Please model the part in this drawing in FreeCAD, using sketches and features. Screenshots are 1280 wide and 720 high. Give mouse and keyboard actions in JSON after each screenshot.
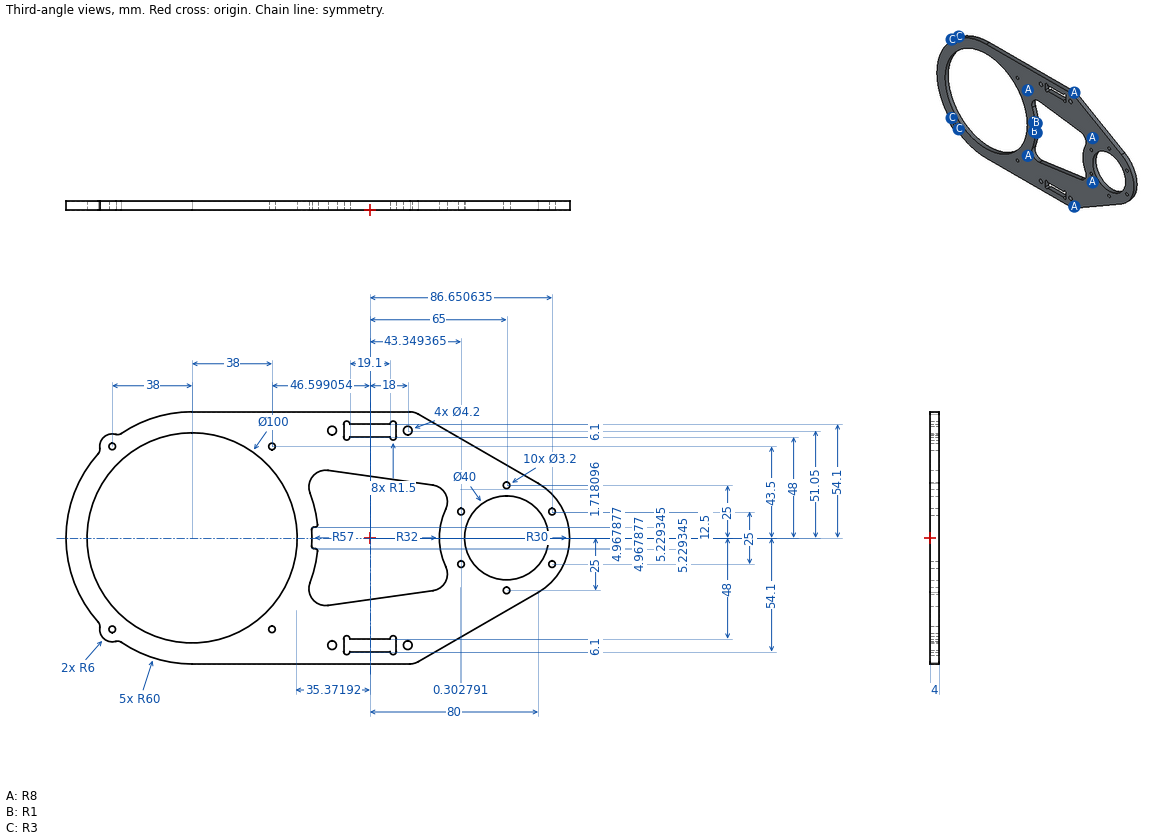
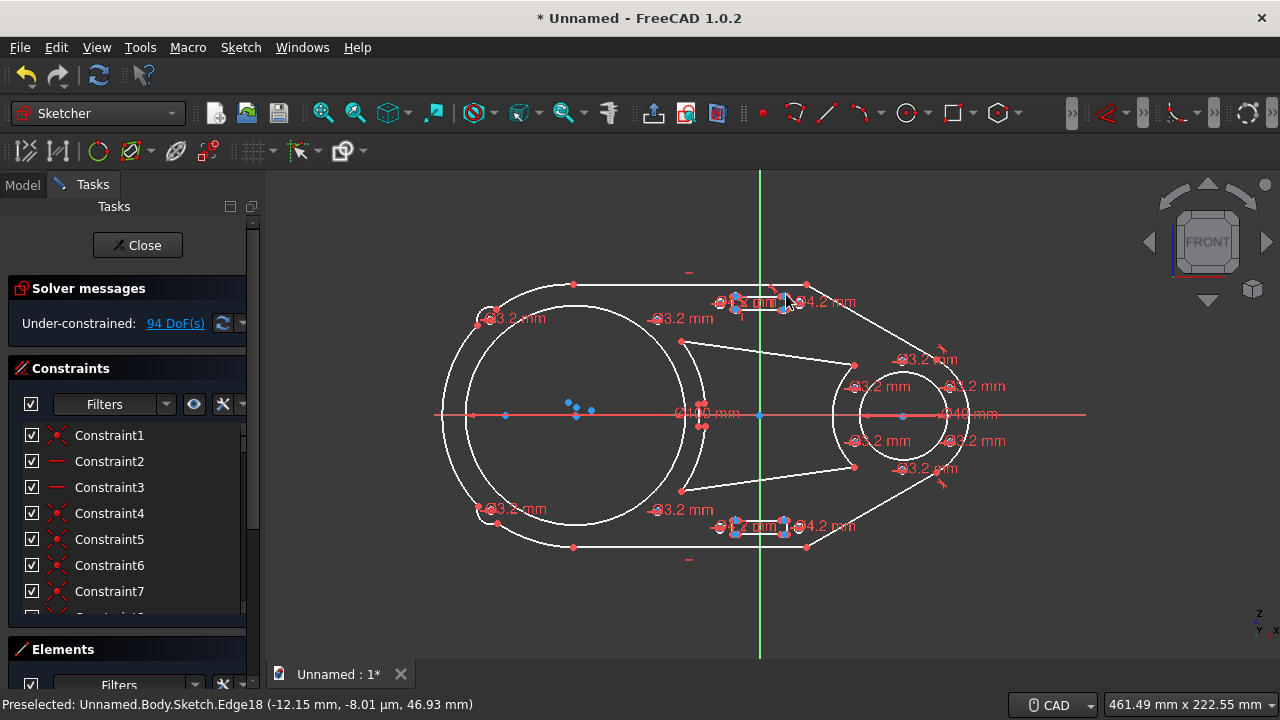
{"action": "scroll", "coordinate": [787, 530], "scroll_direction": "up", "scroll_amount": 7}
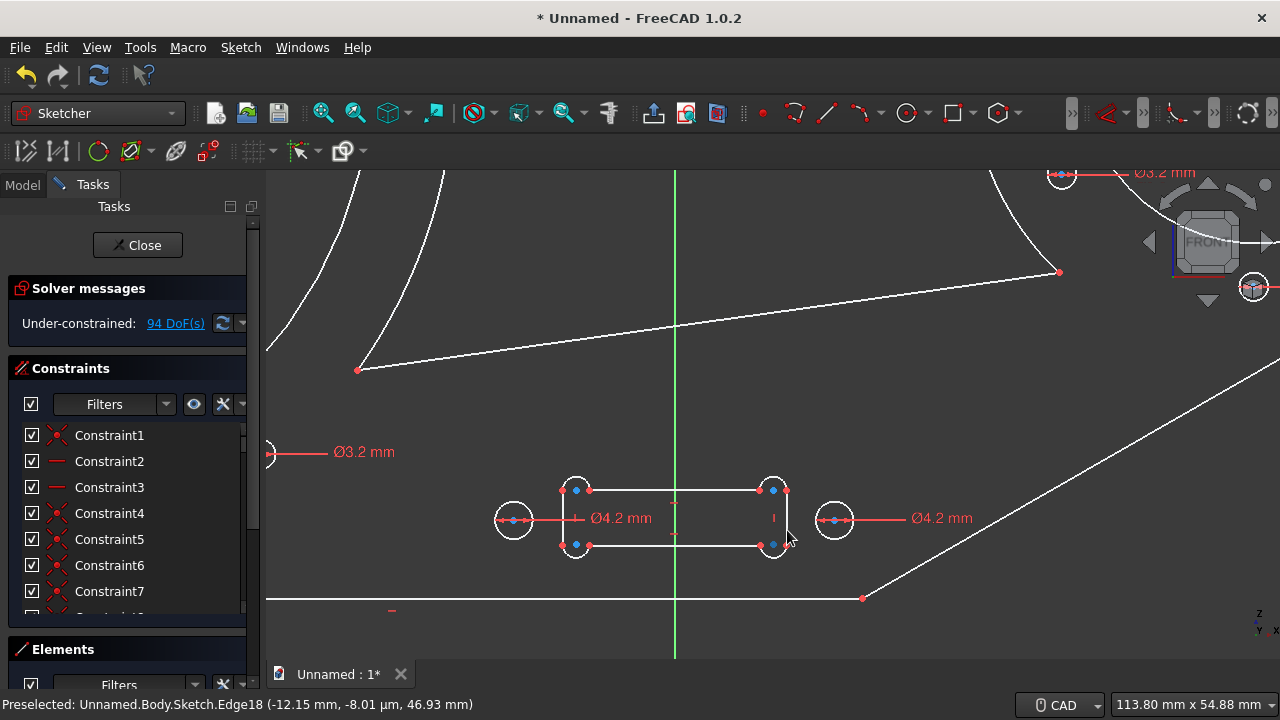
{"action": "left_click", "coordinate": [787, 529]}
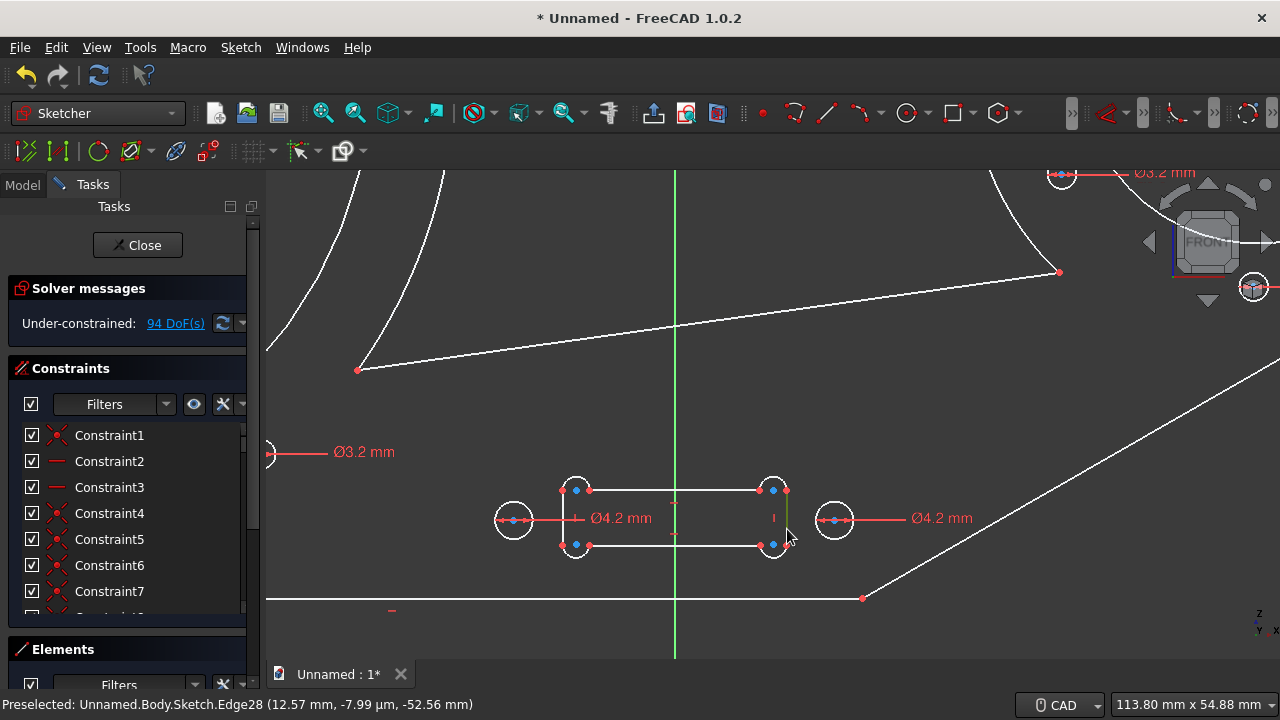
{"action": "left_click", "coordinate": [766, 556]}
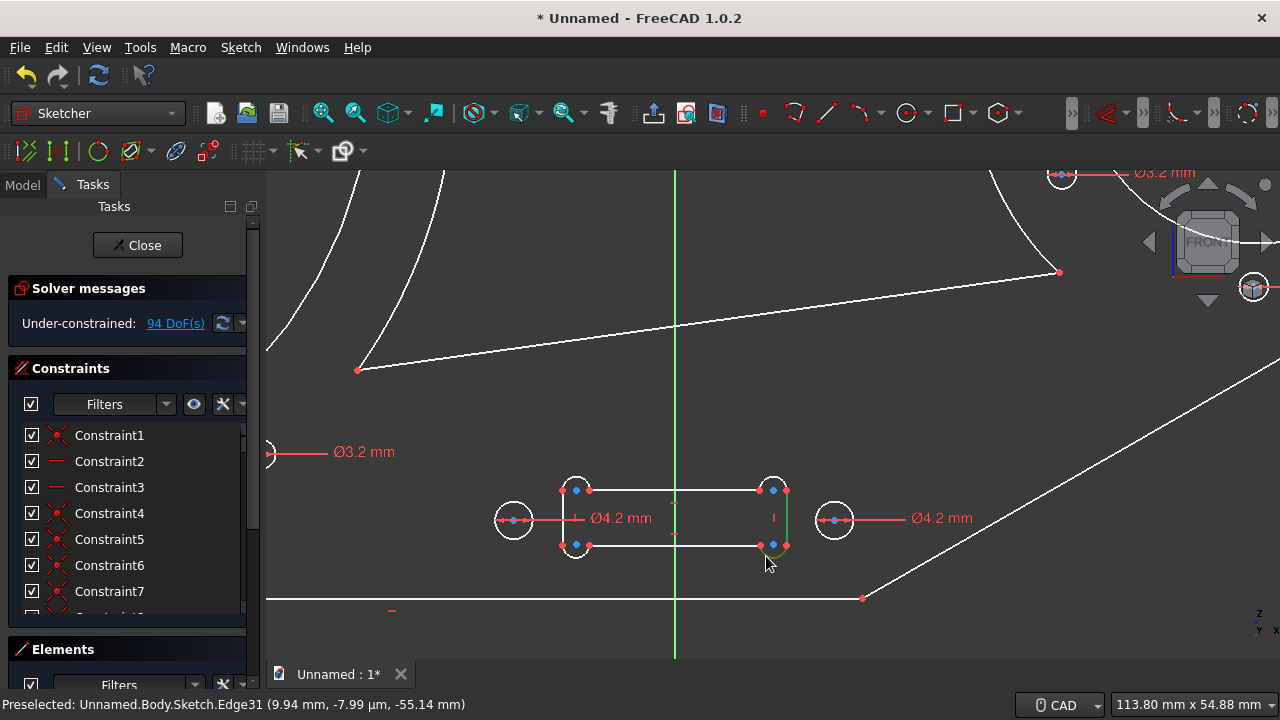
{"action": "key", "text": "t"}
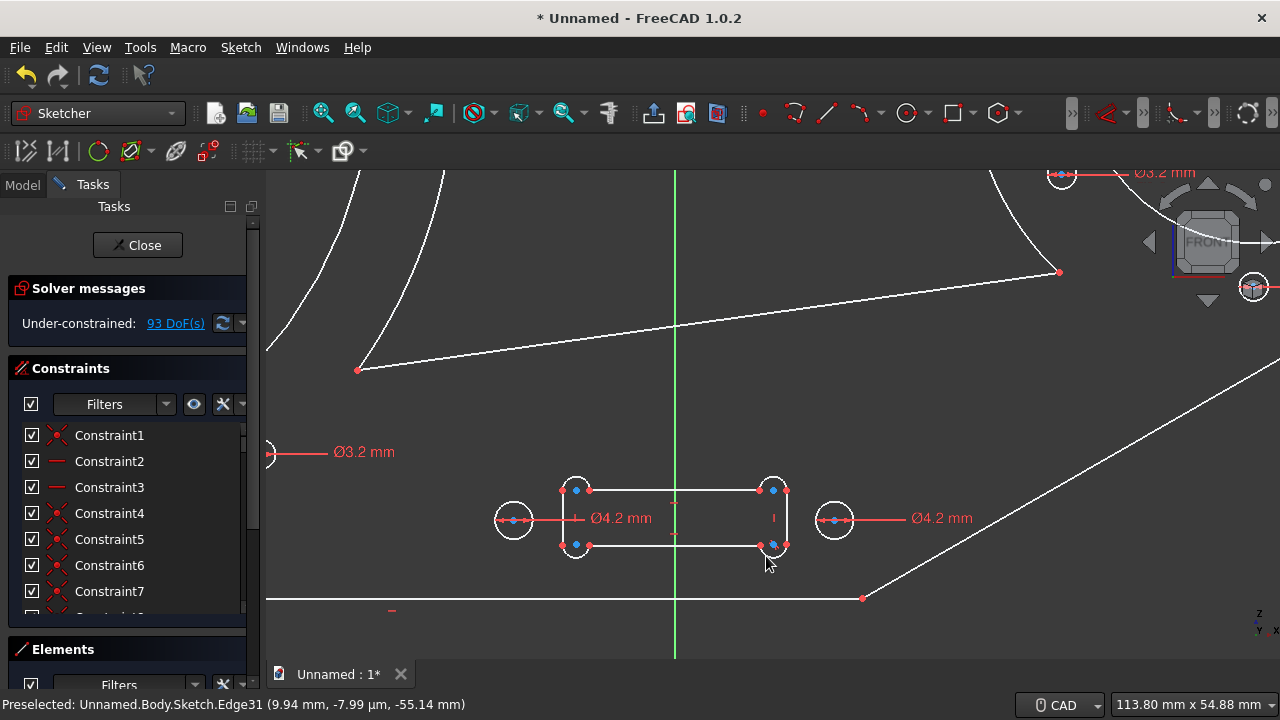
{"action": "left_click", "coordinate": [787, 528]}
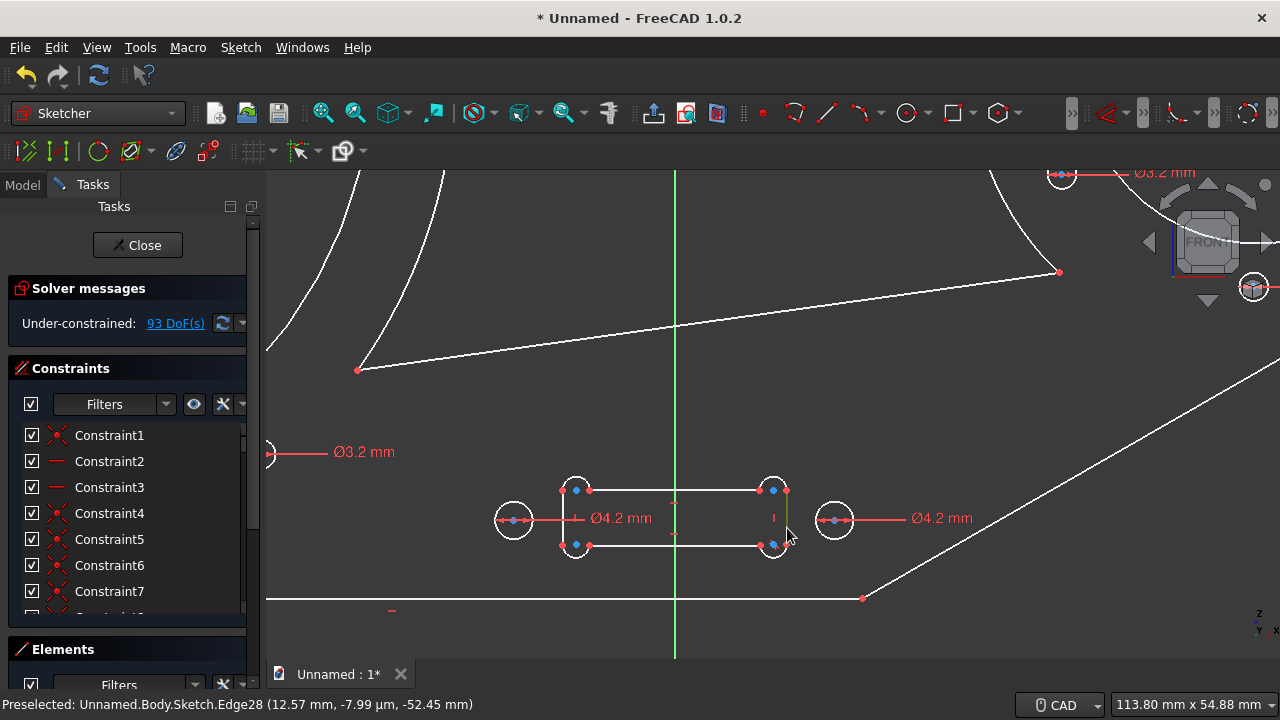
{"action": "left_click", "coordinate": [781, 479]}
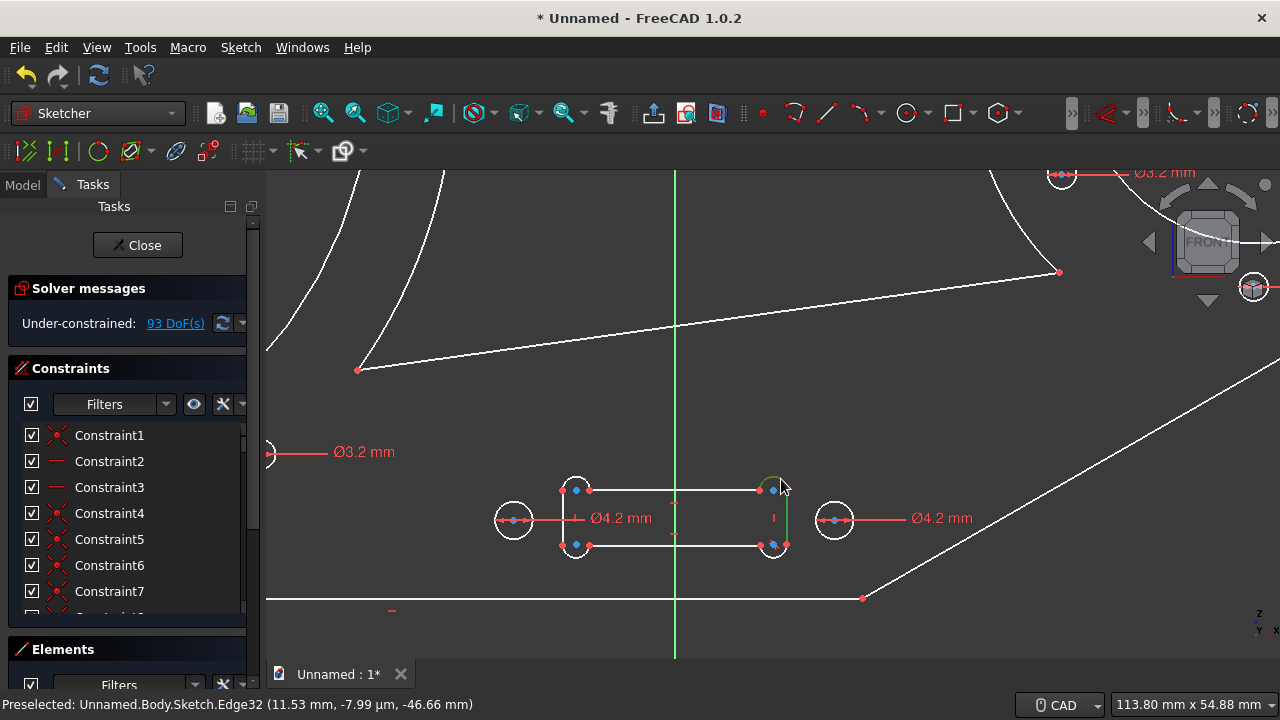
{"action": "key", "text": "t"}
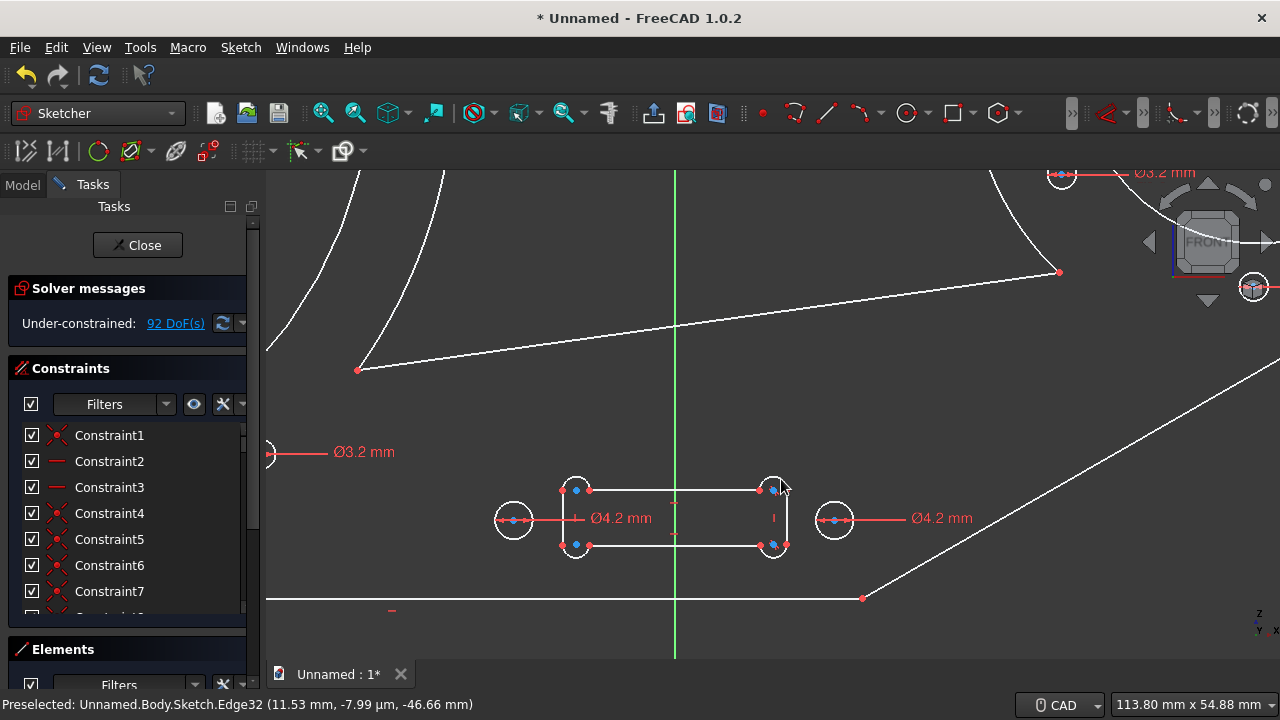
{"action": "left_click", "coordinate": [563, 507]}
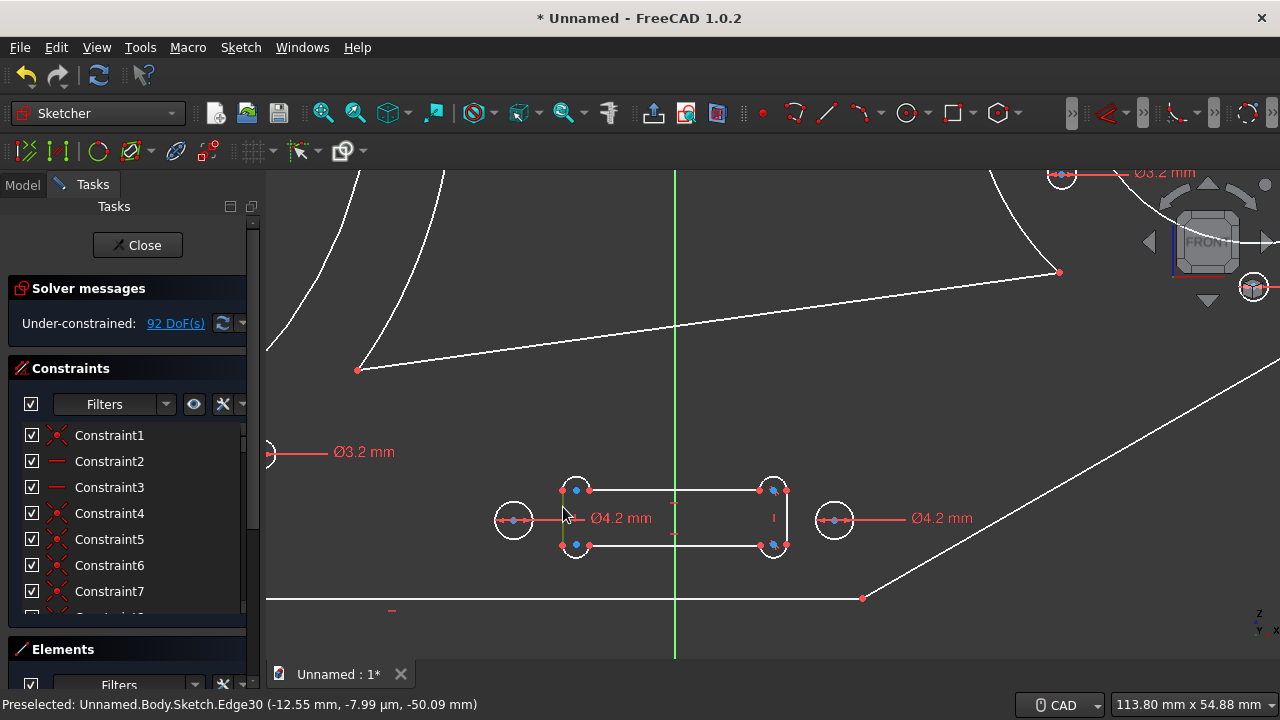
{"action": "left_click", "coordinate": [584, 479]}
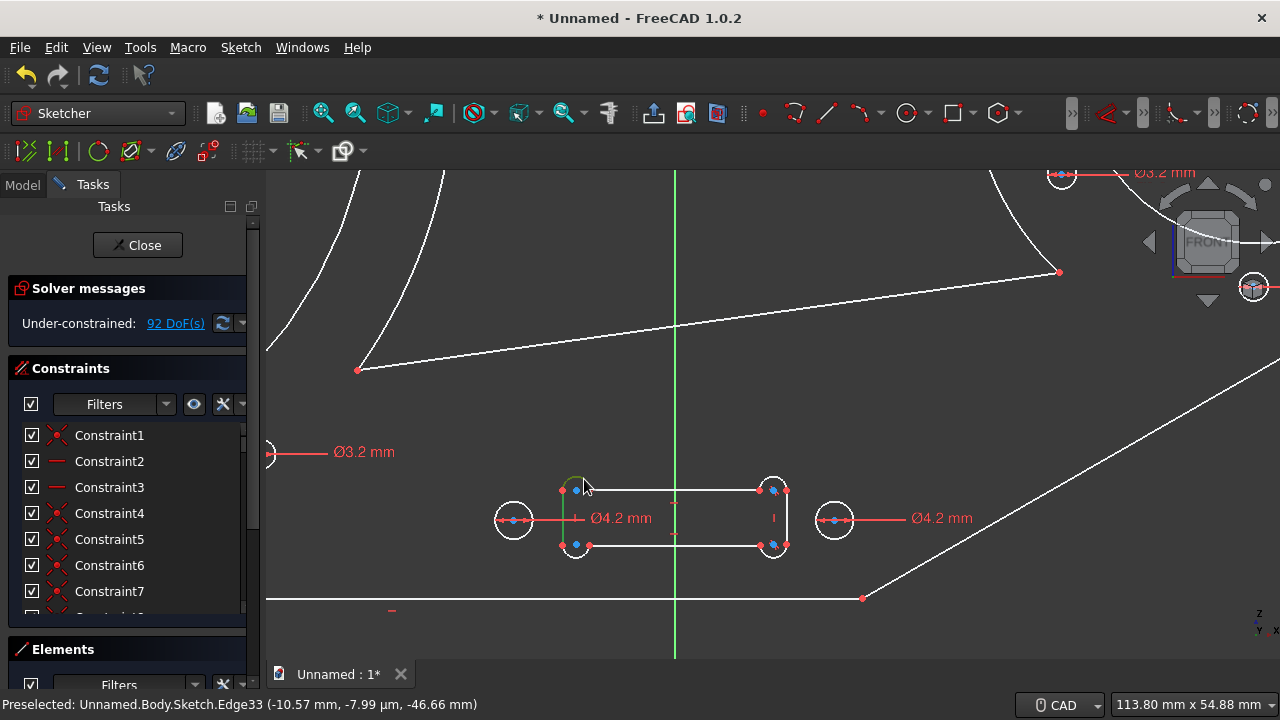
{"action": "key", "text": "t"}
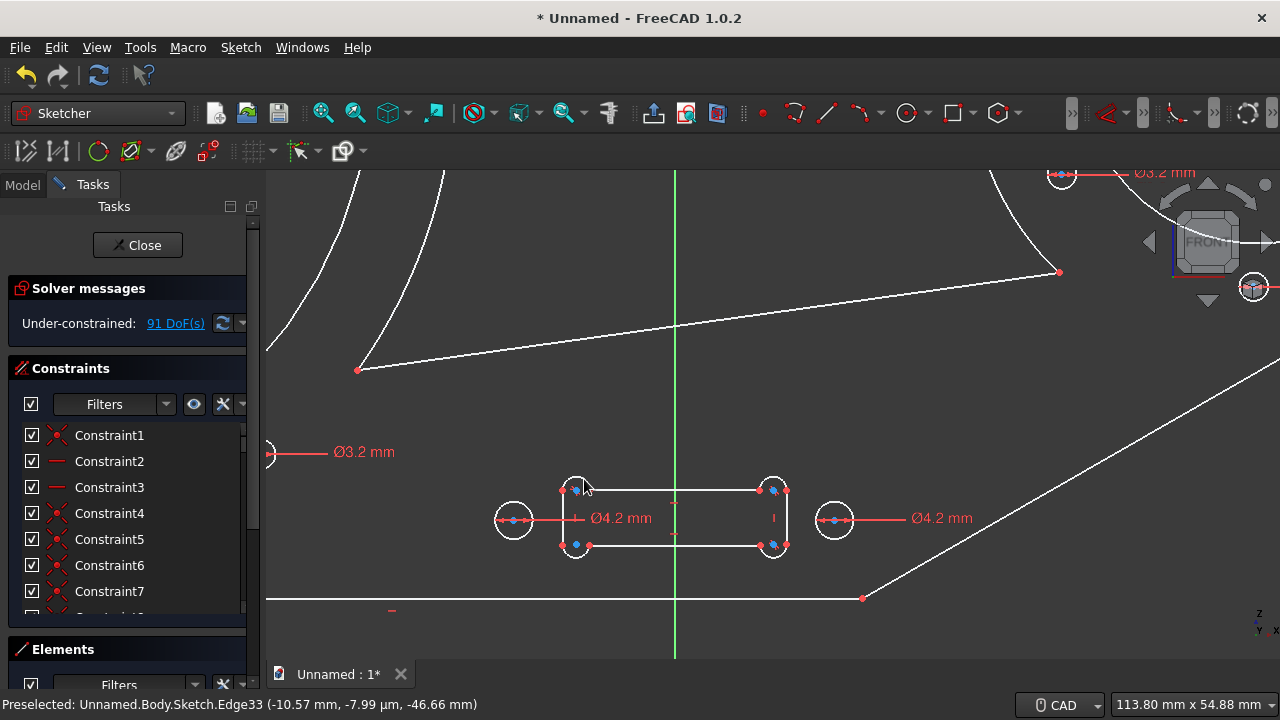
{"action": "left_click", "coordinate": [563, 507]}